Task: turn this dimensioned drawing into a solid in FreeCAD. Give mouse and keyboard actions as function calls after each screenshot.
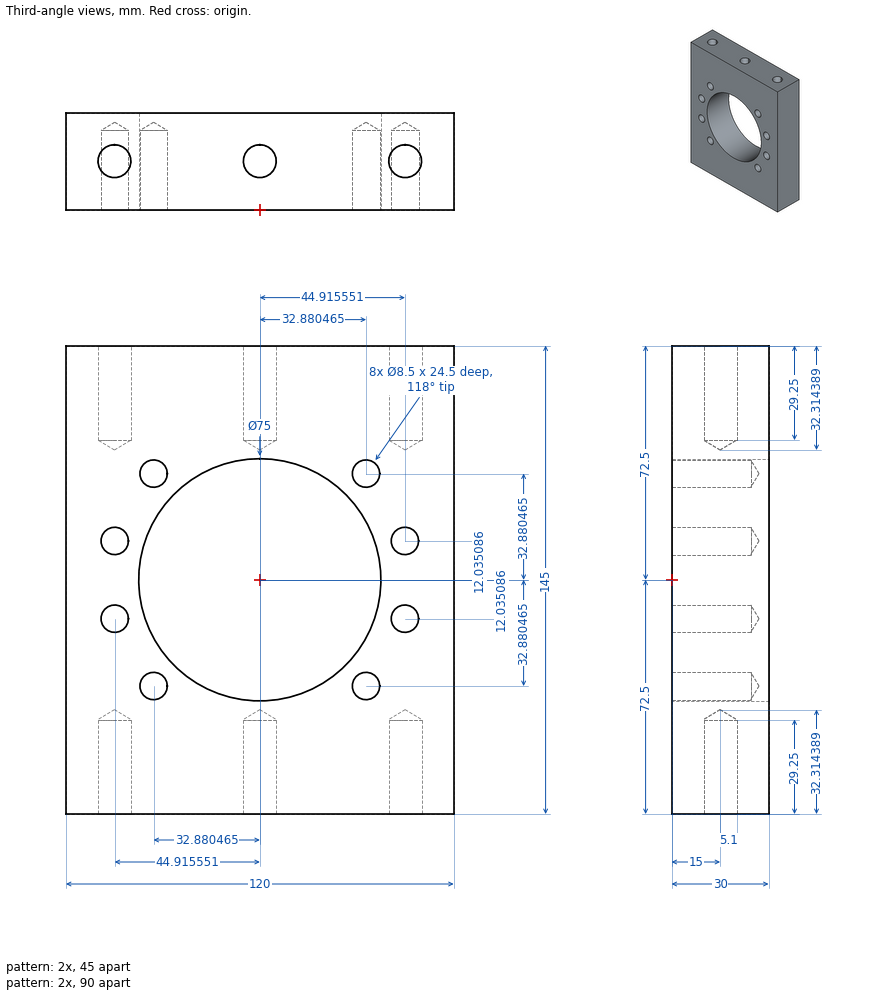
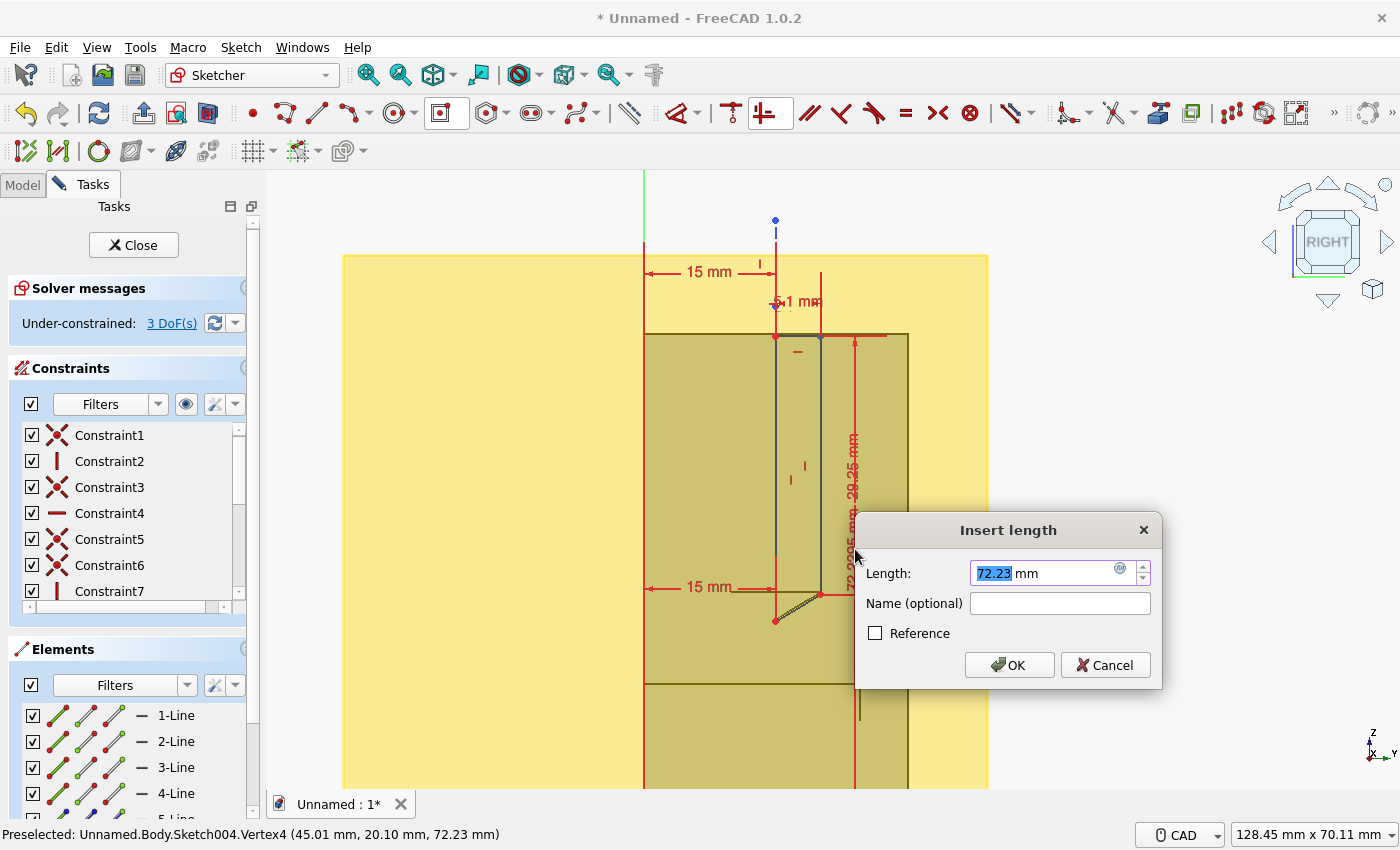
text(72.5)
key(Return)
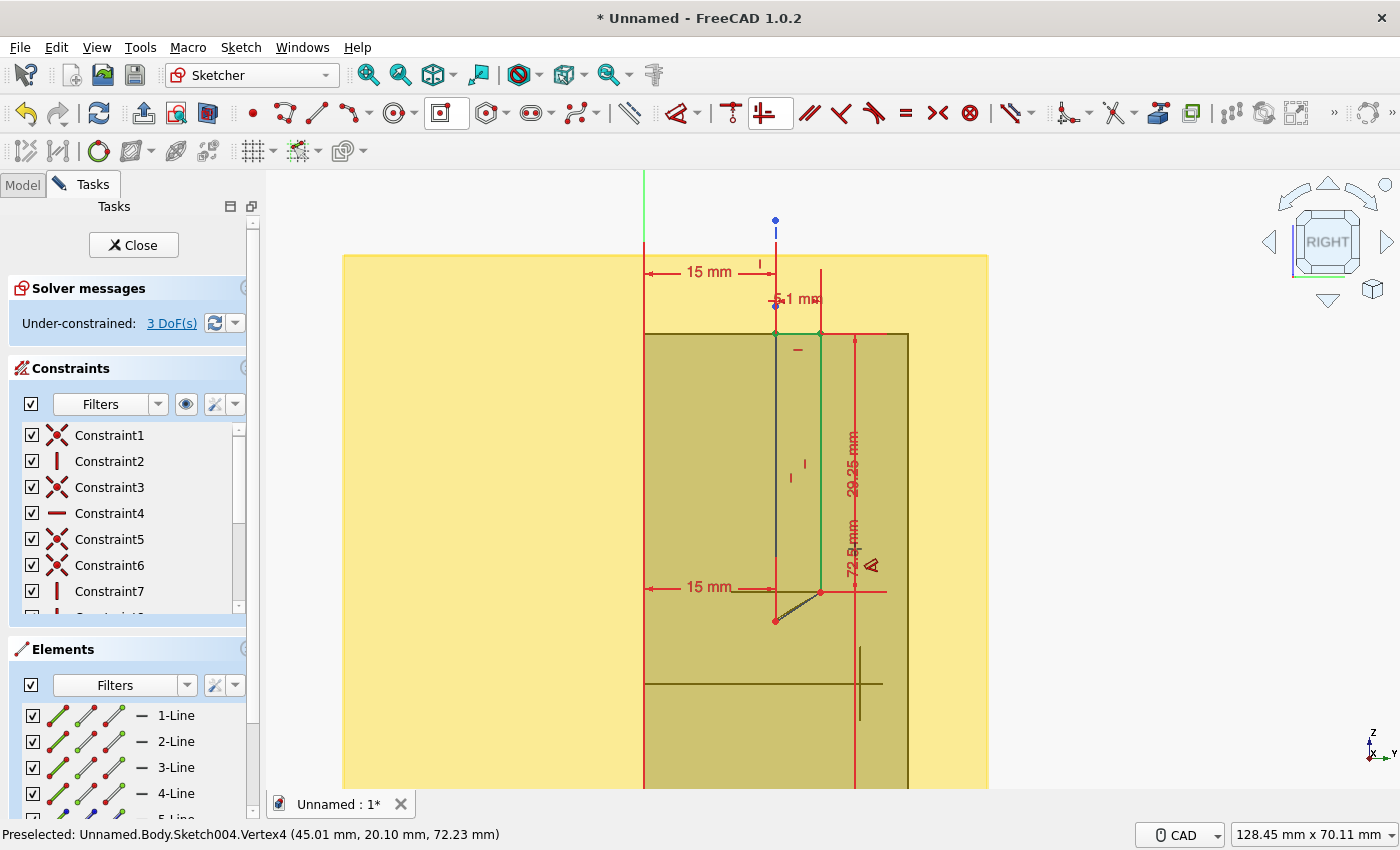
click(776, 420)
click(742, 478)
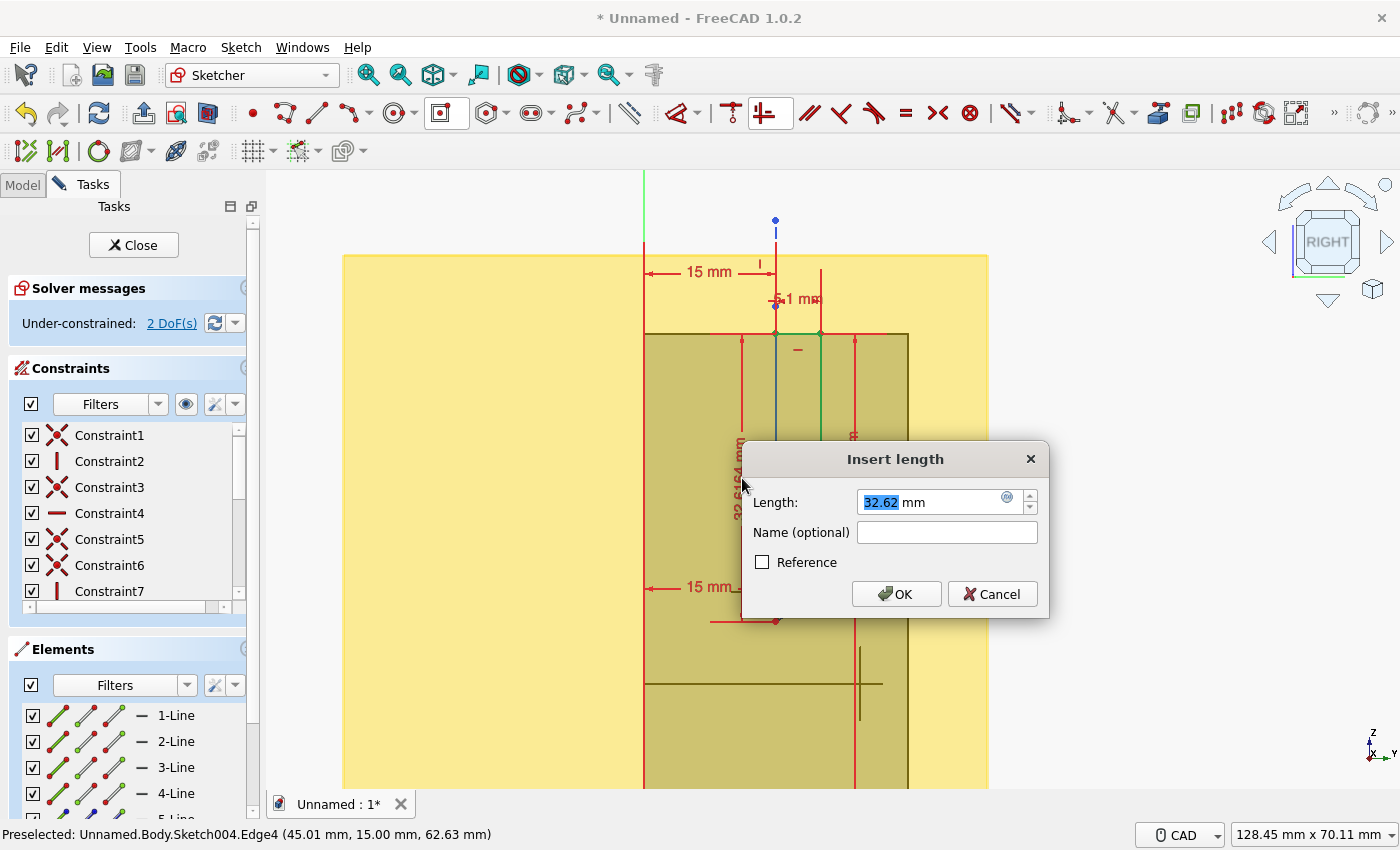
text(32.314389)
key(Return)
key(Escape)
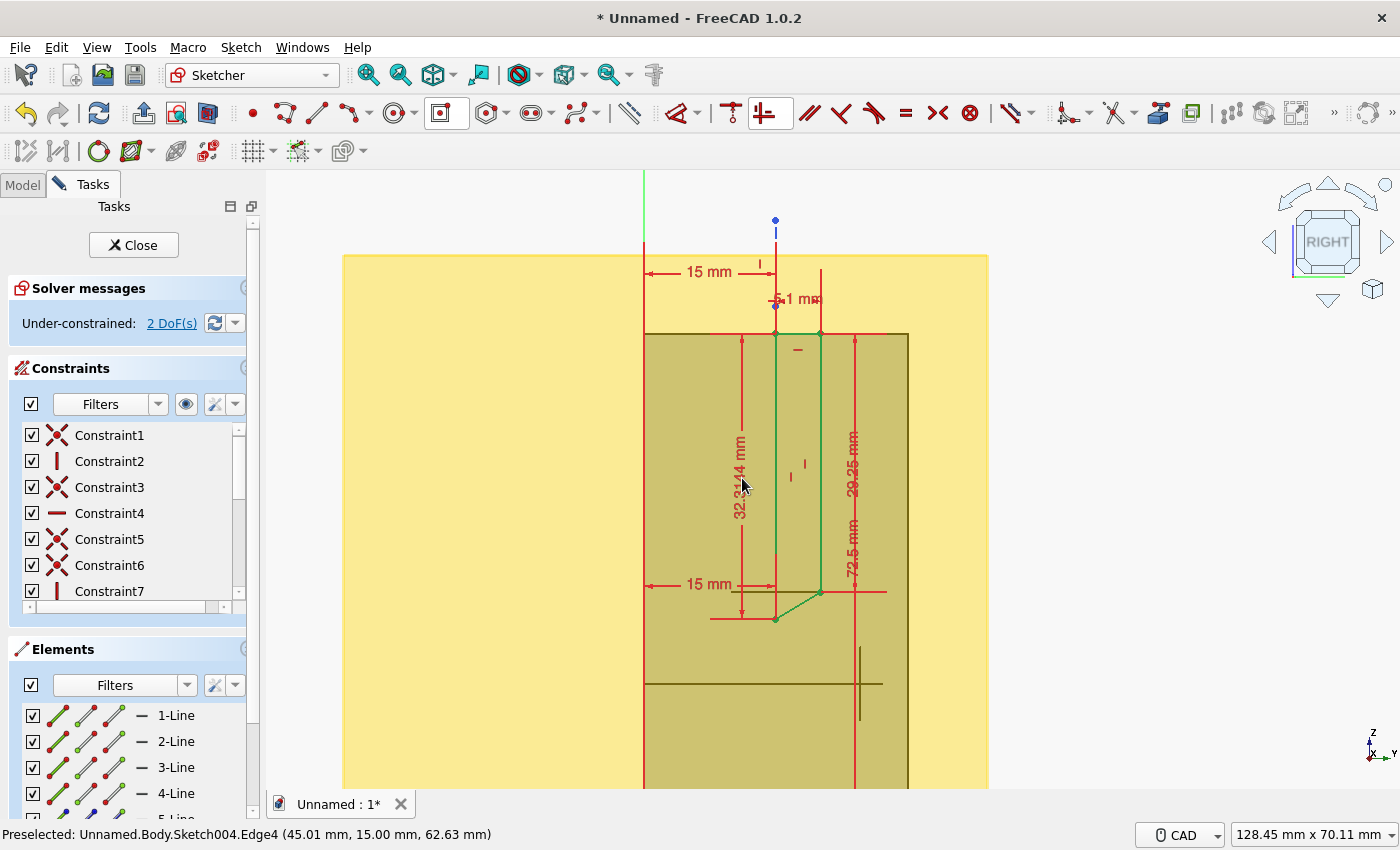
click(134, 245)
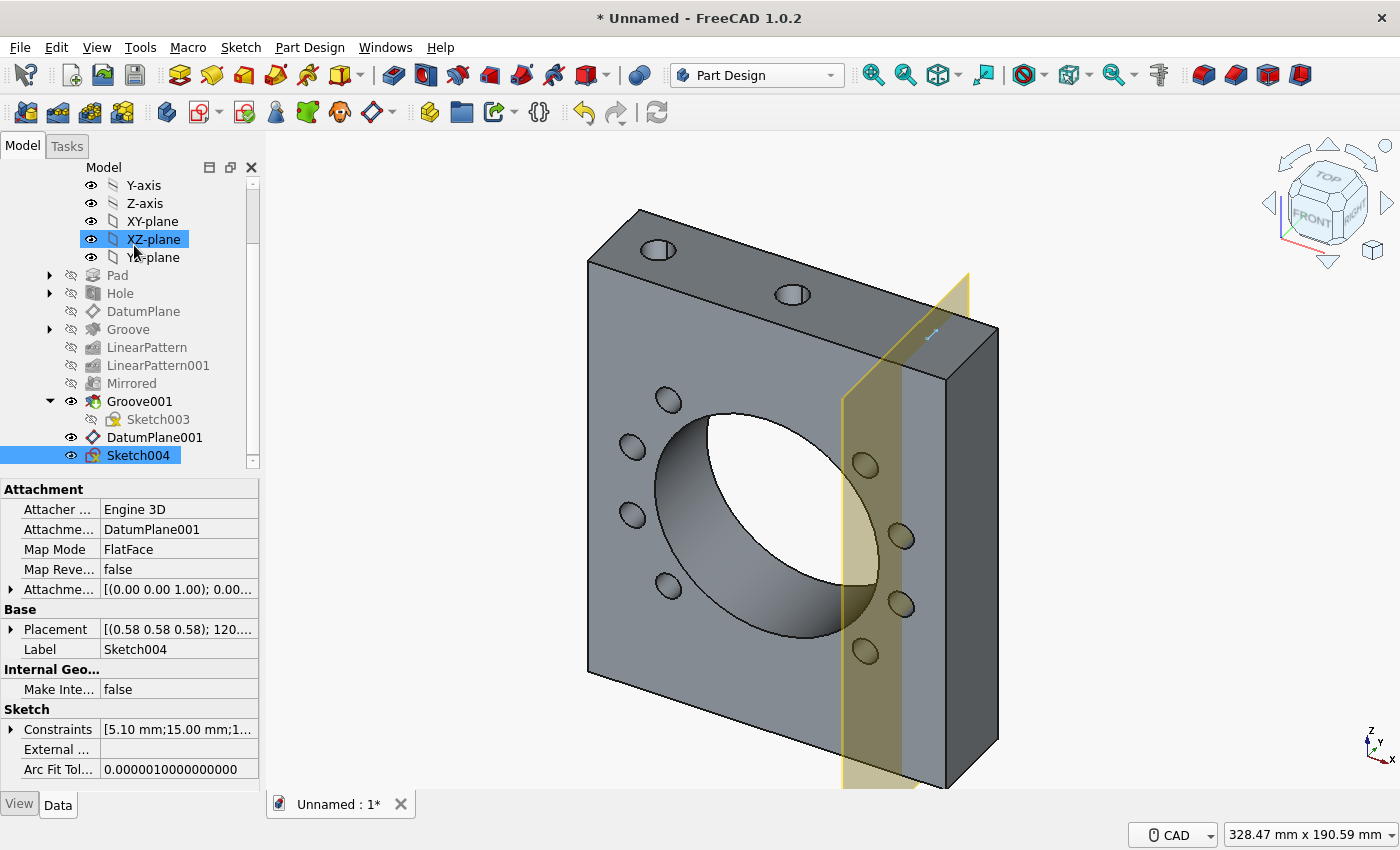
click(458, 76)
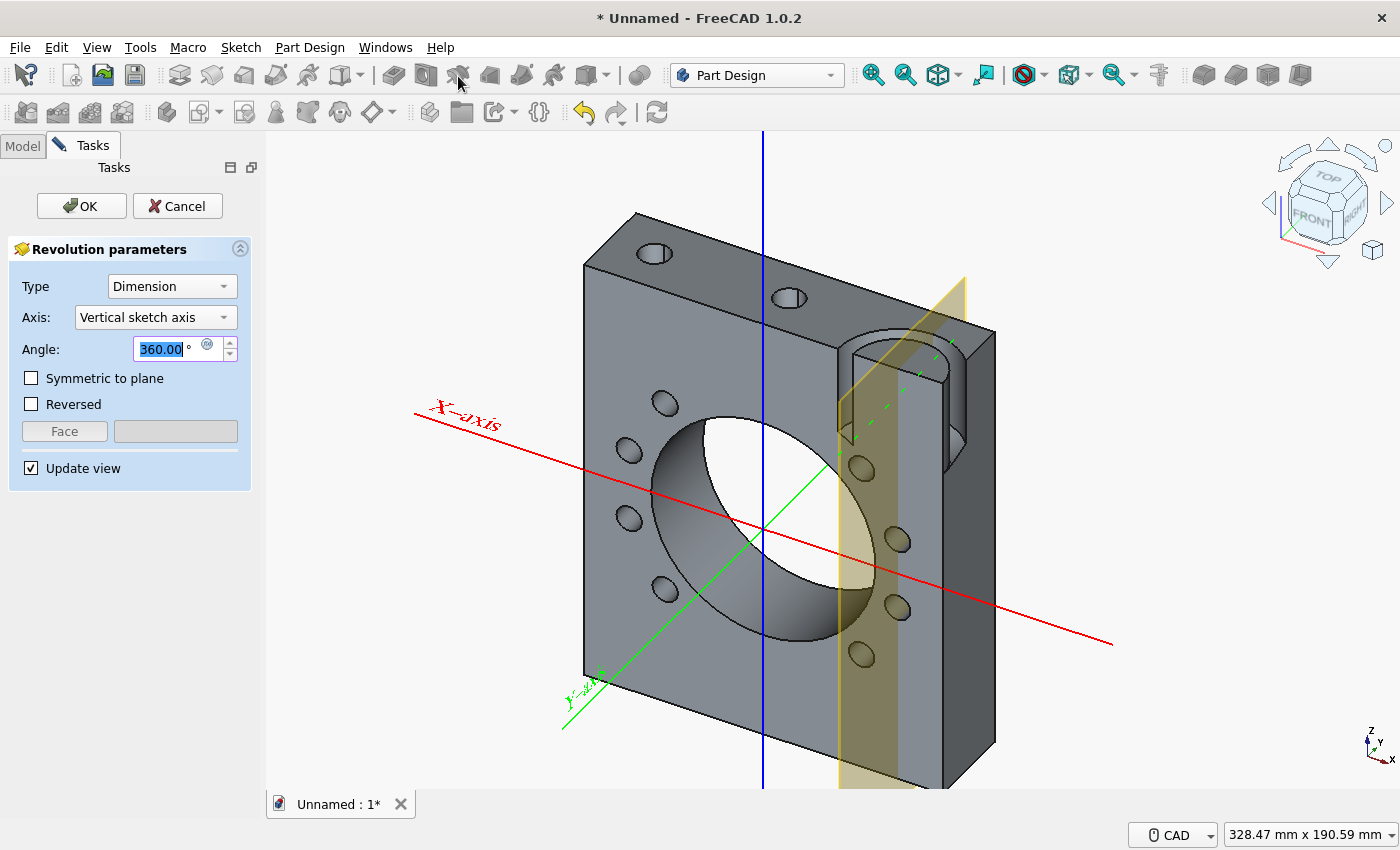
click(156, 318)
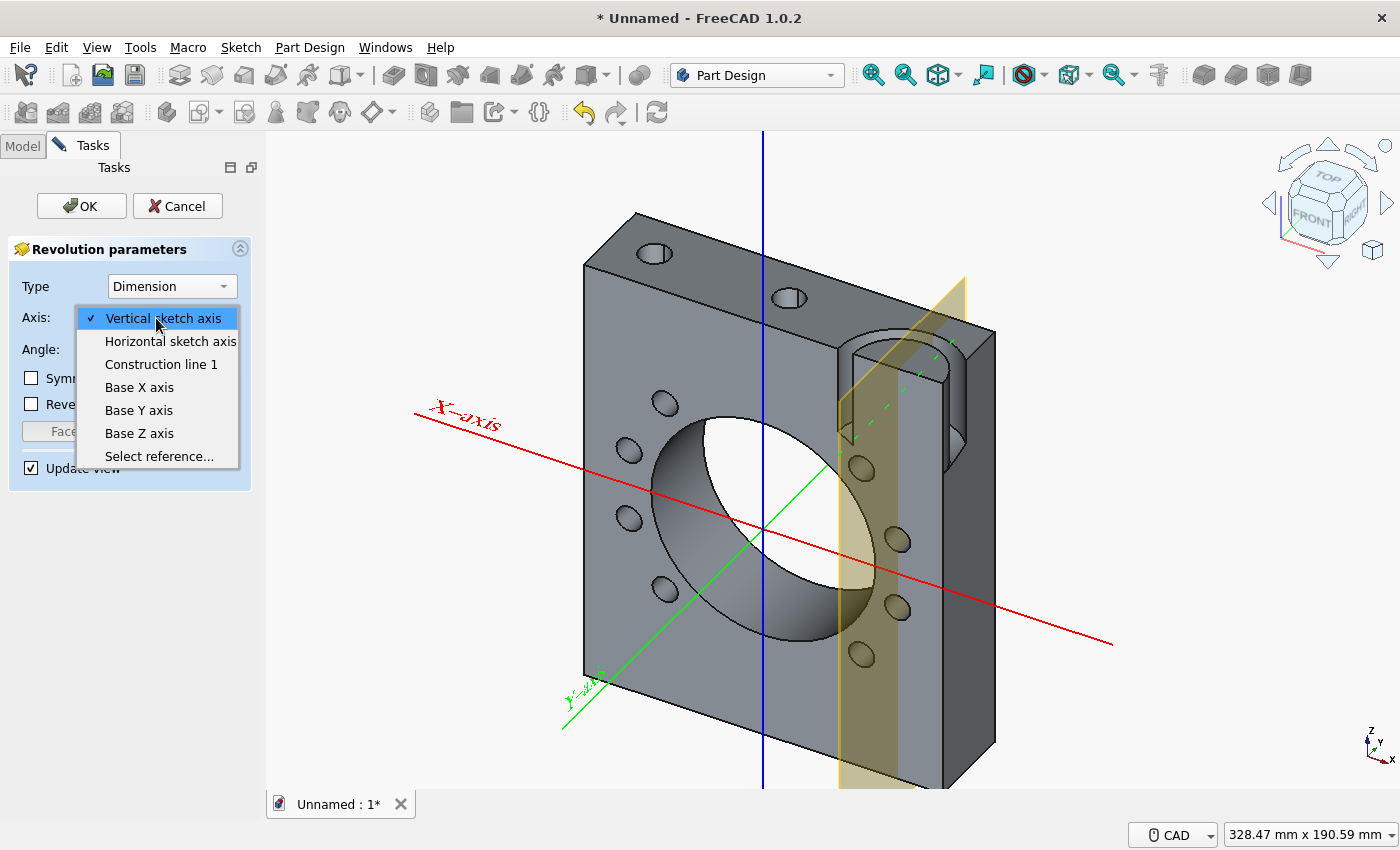
click(156, 364)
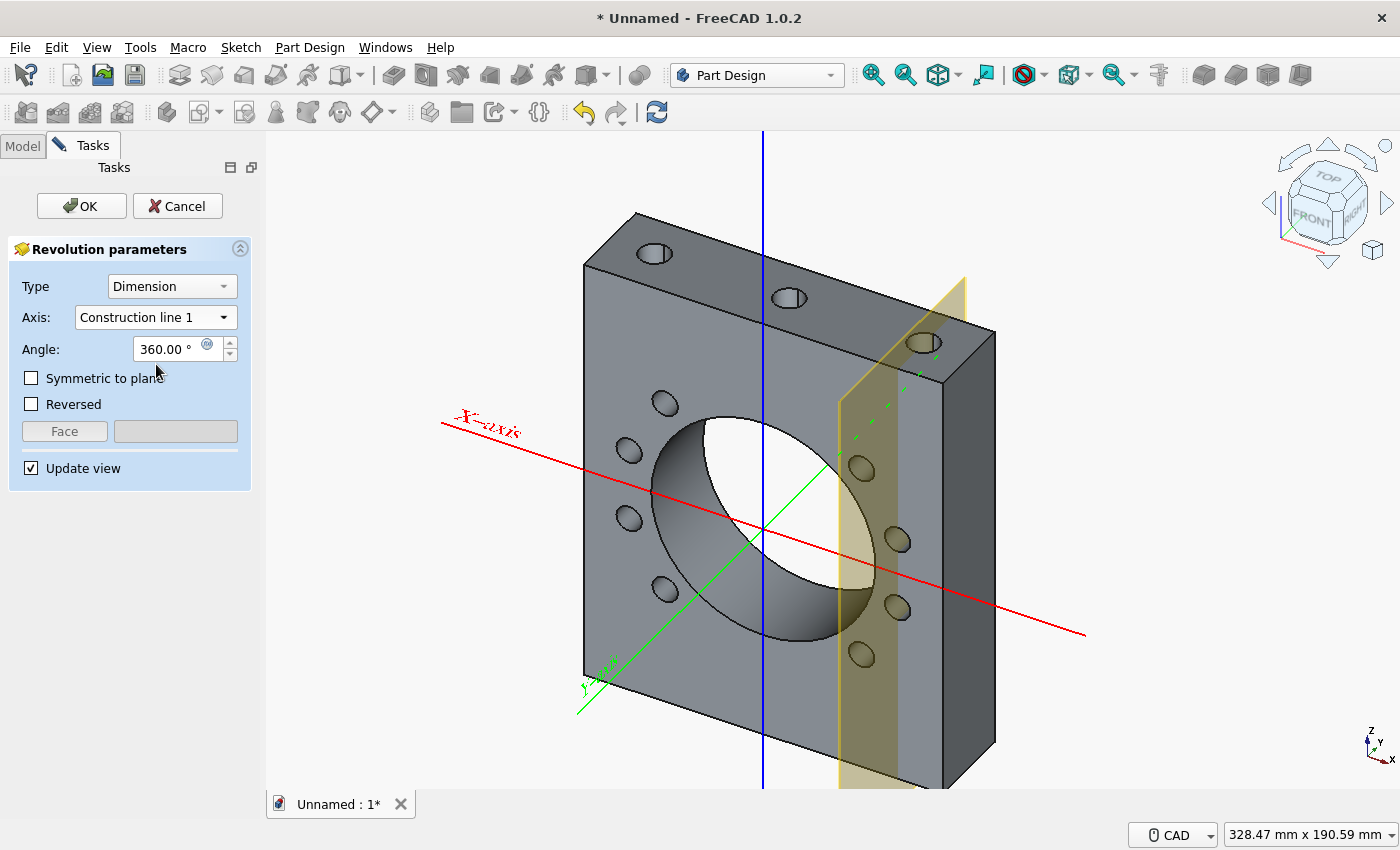
click(82, 206)